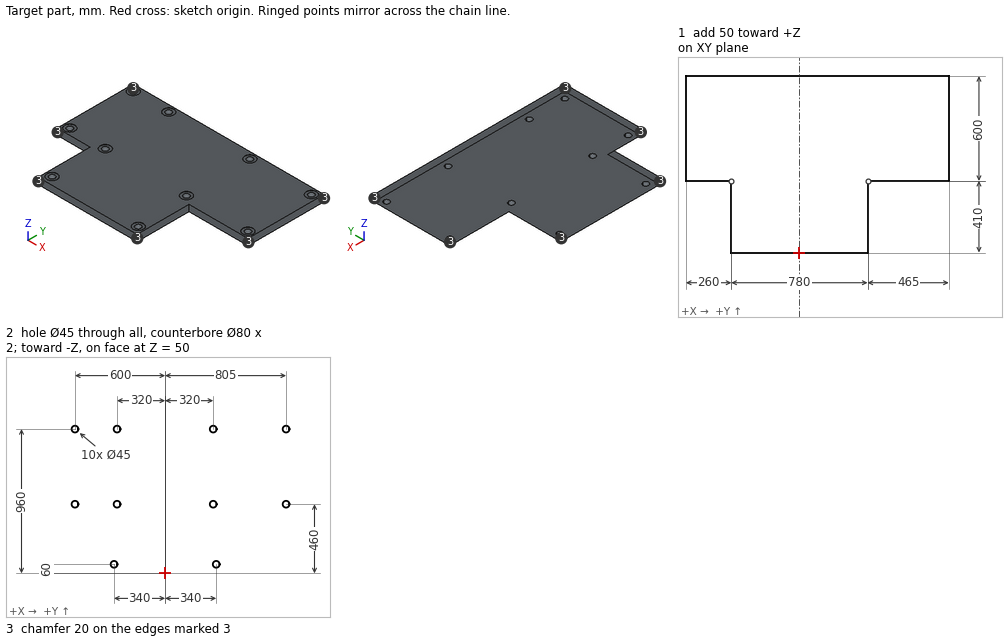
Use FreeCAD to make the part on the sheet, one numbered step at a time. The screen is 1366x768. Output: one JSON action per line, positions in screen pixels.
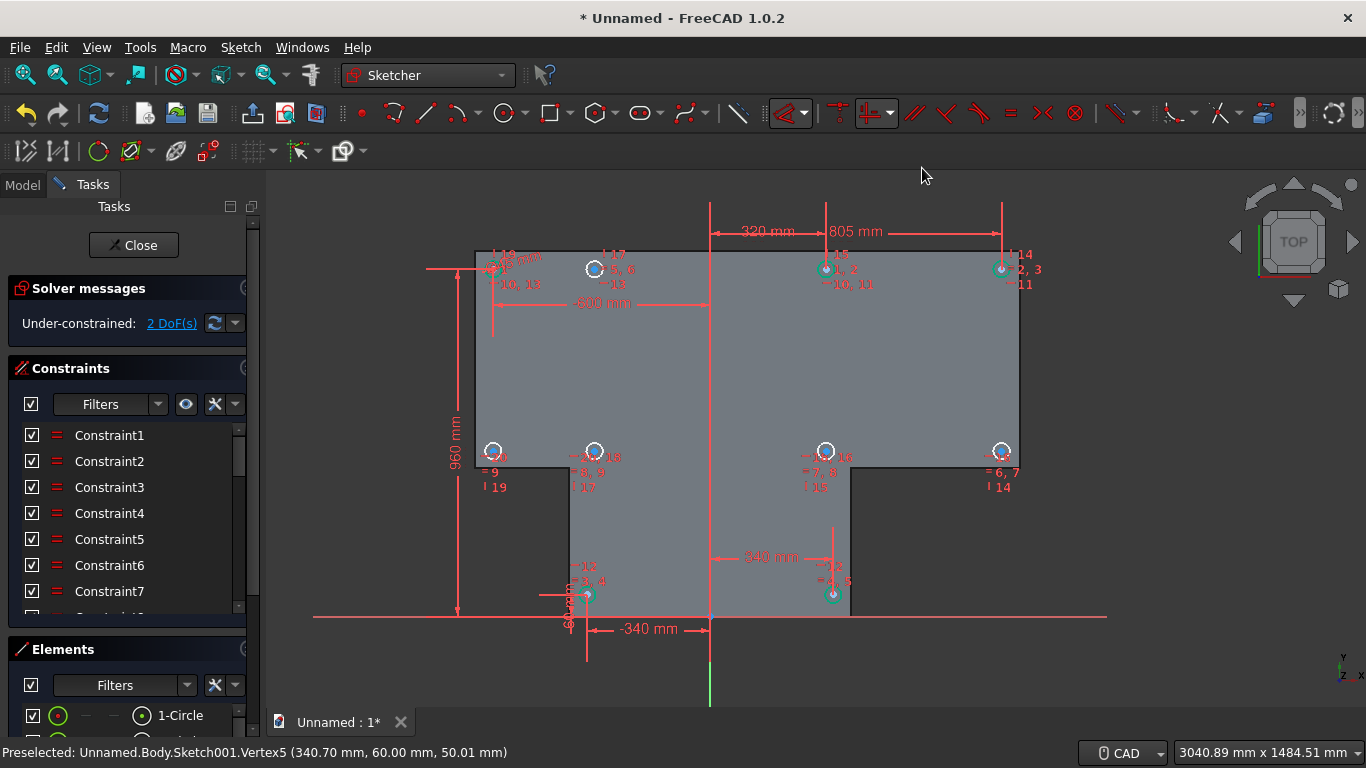
{"action": "left_click", "coordinate": [595, 269]}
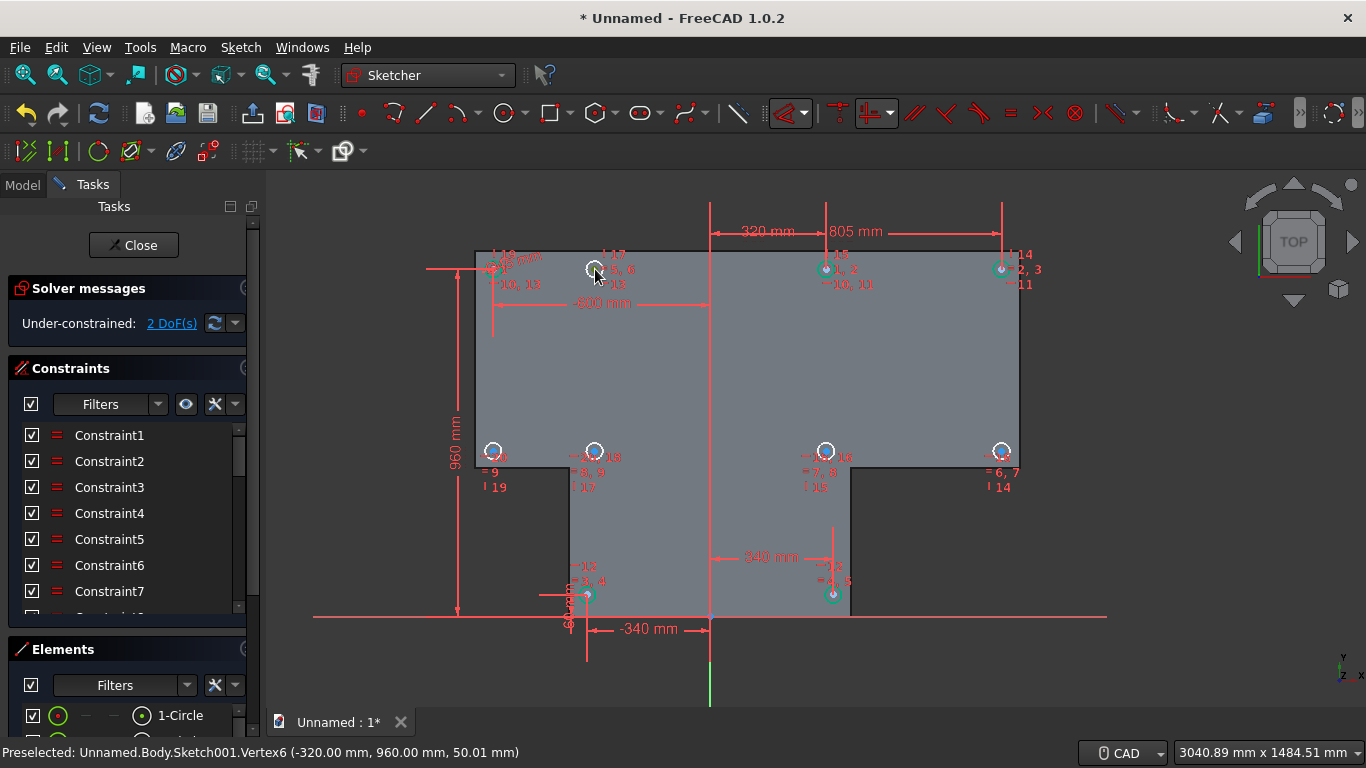
{"action": "left_click", "coordinate": [806, 114]}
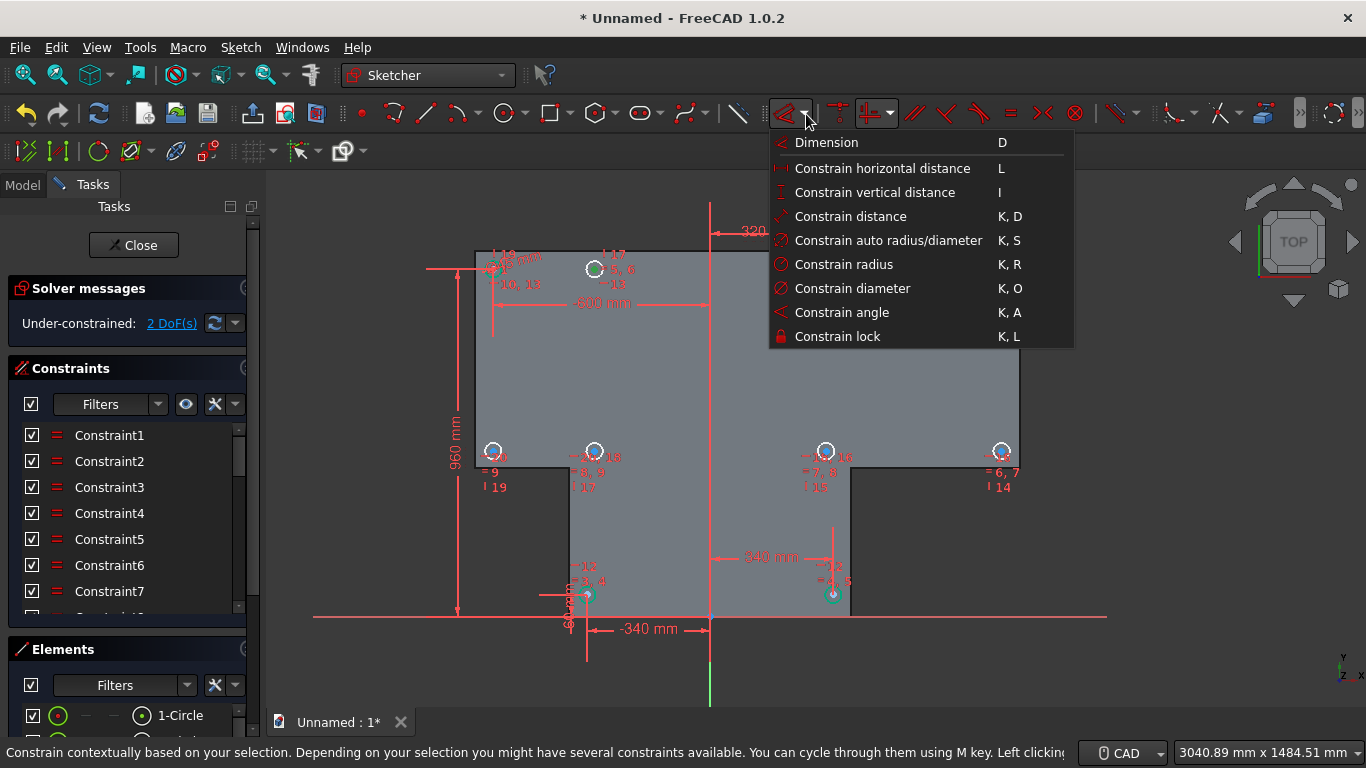
{"action": "left_click", "coordinate": [922, 168]}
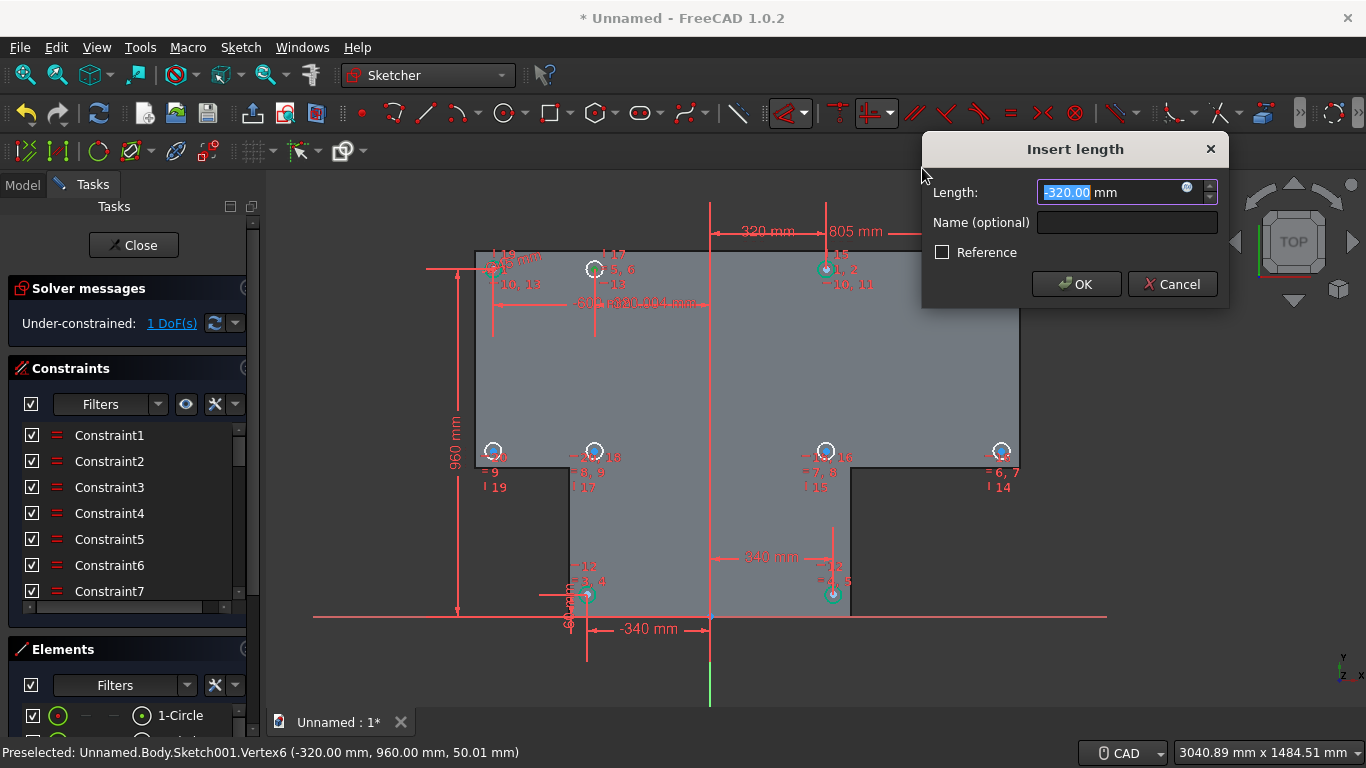
{"action": "type", "text": "-320"}
{"action": "key", "text": "Return"}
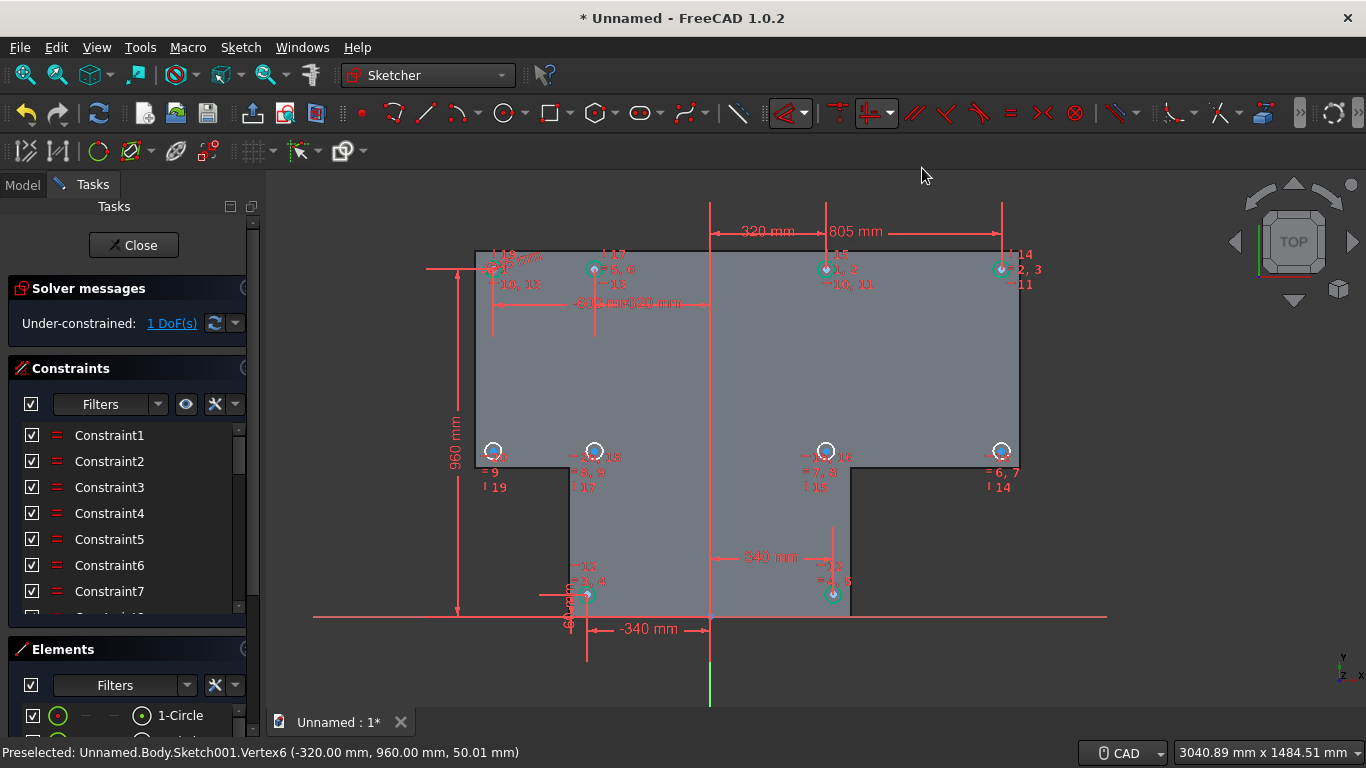
{"action": "left_click", "coordinate": [1002, 451]}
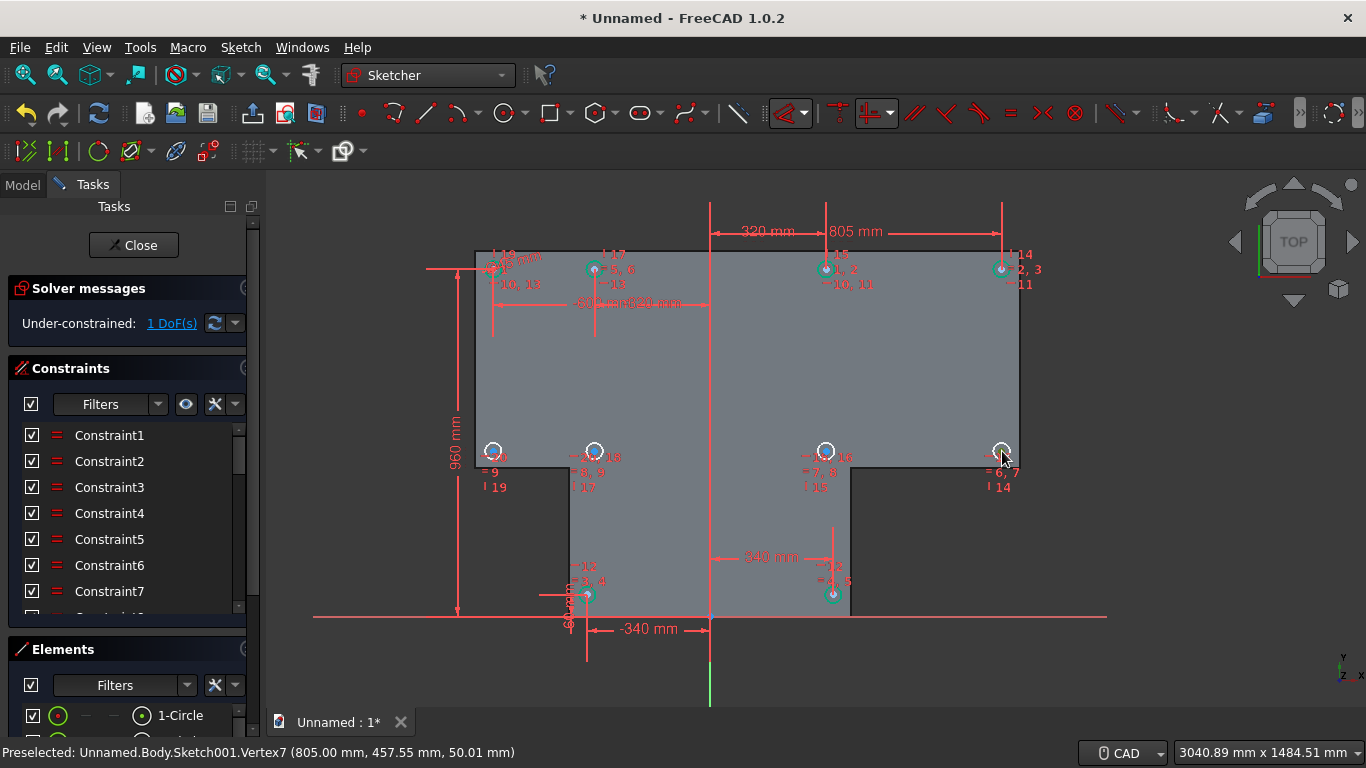
{"action": "key", "text": "i"}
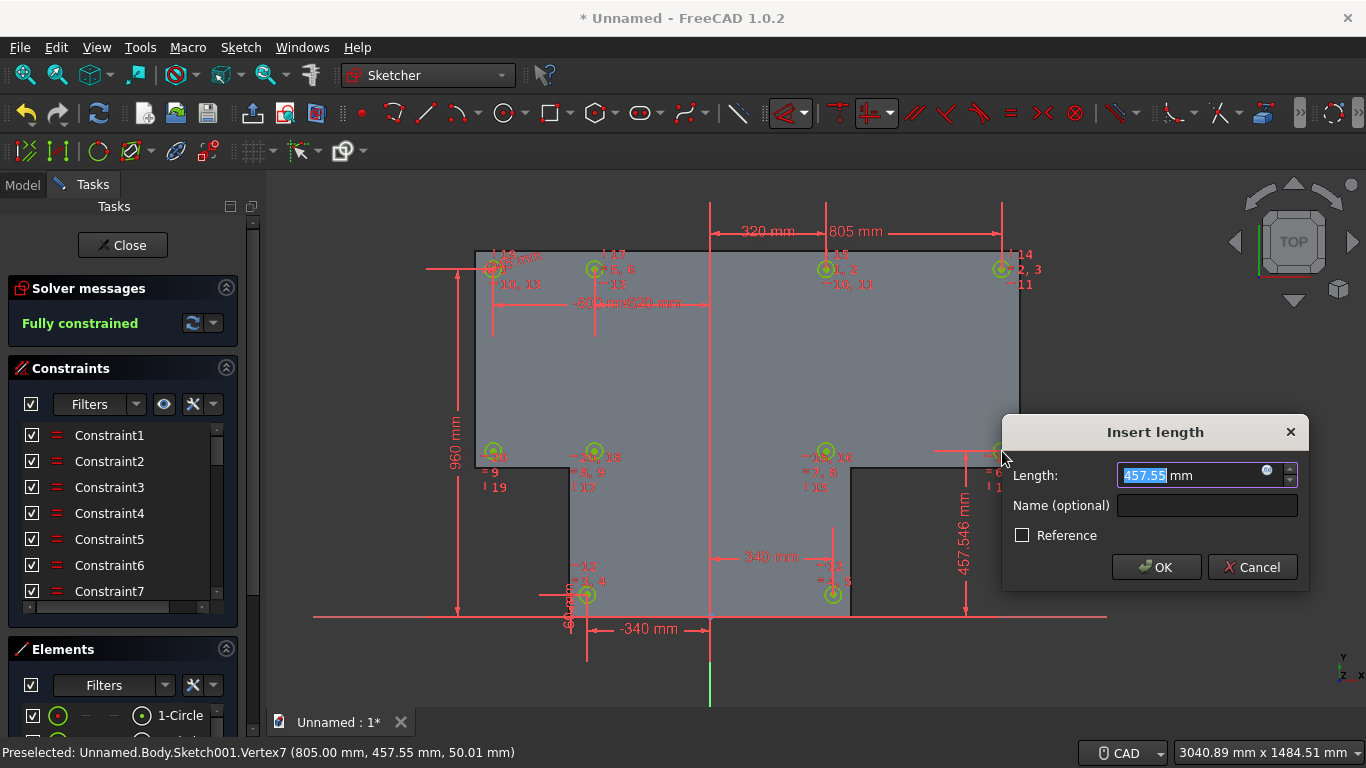
{"action": "type", "text": "460"}
{"action": "key", "text": "Return"}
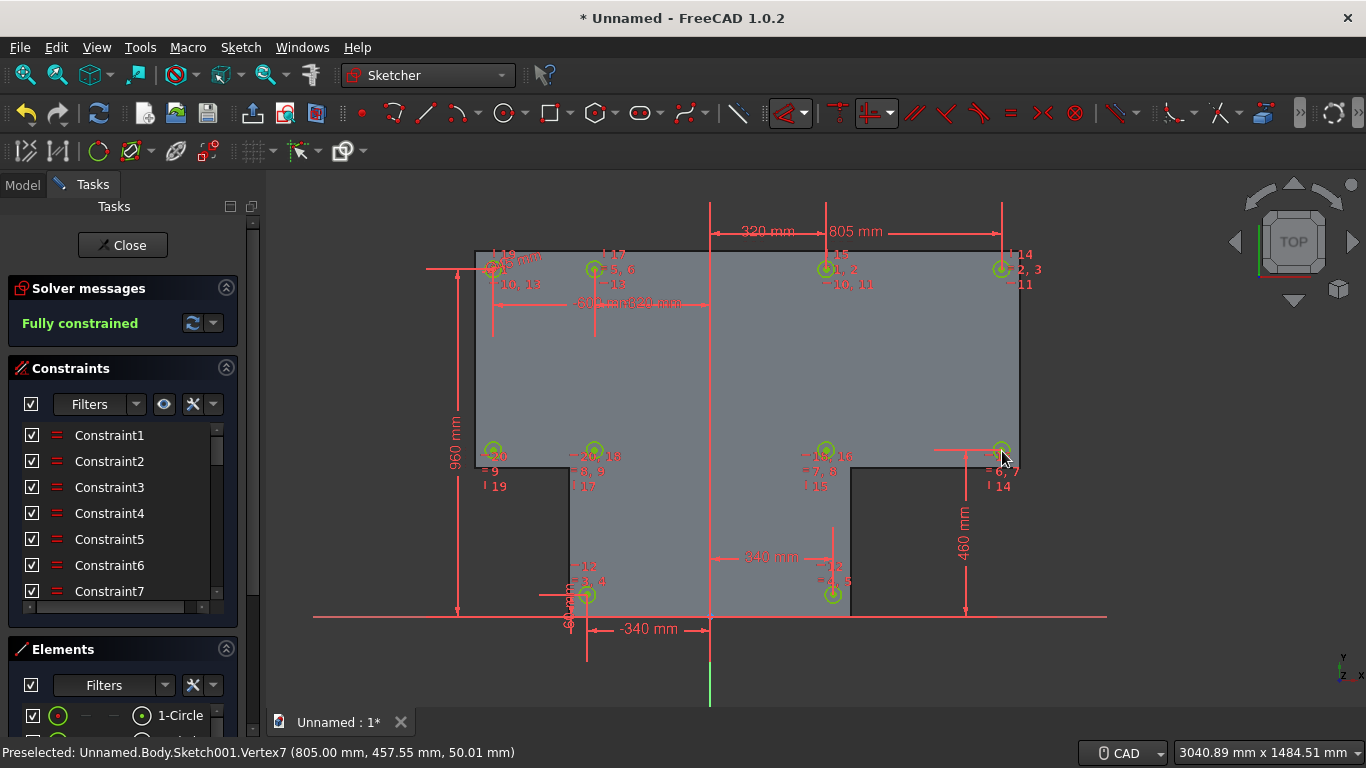
{"action": "left_click", "coordinate": [123, 245]}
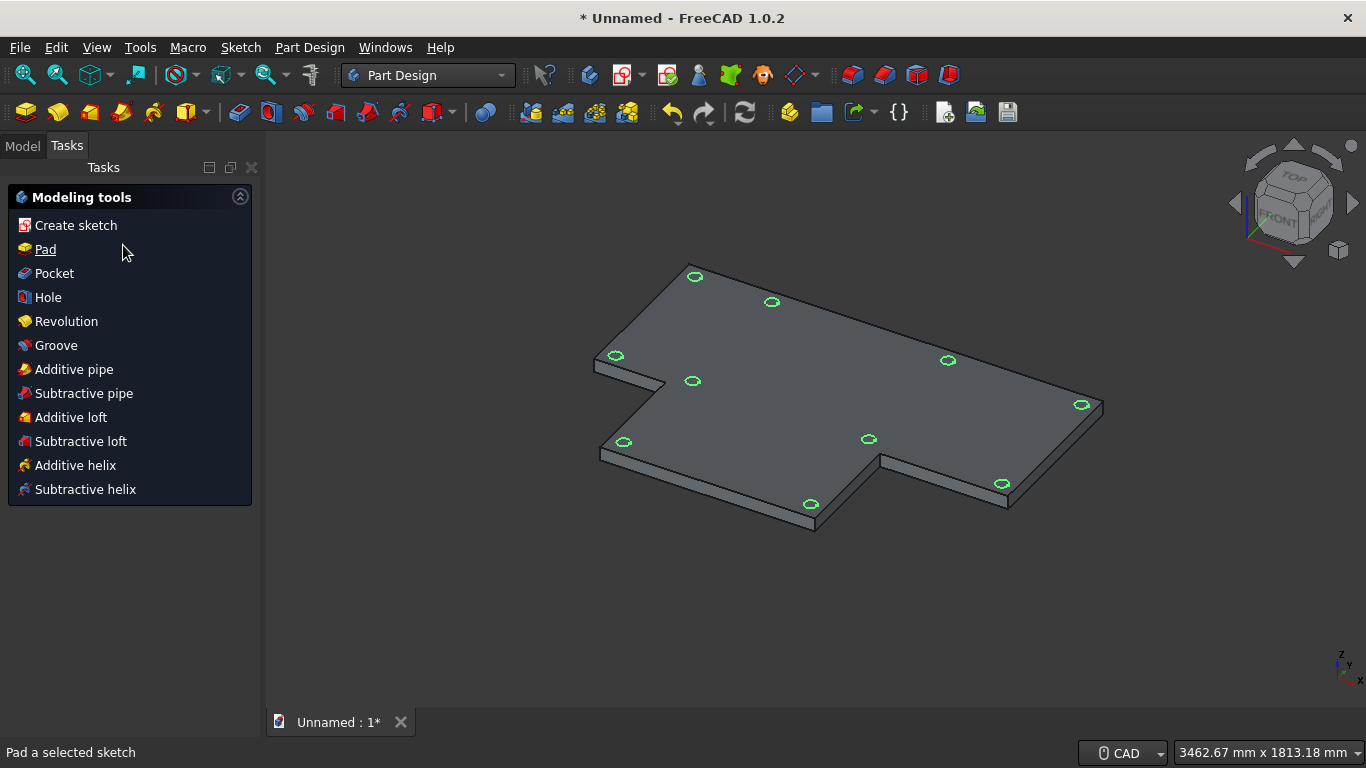
{"action": "left_click", "coordinate": [272, 112]}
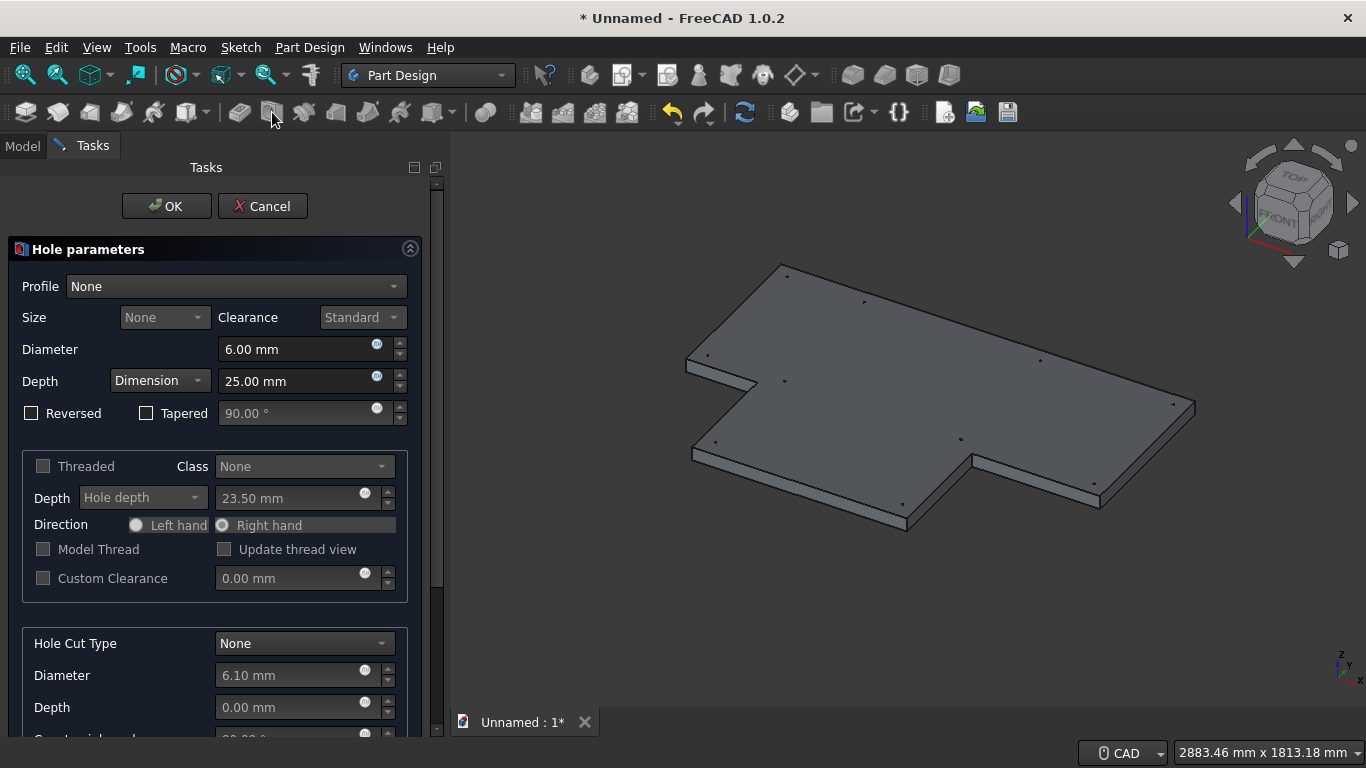
{"action": "triple_click", "coordinate": [305, 349]}